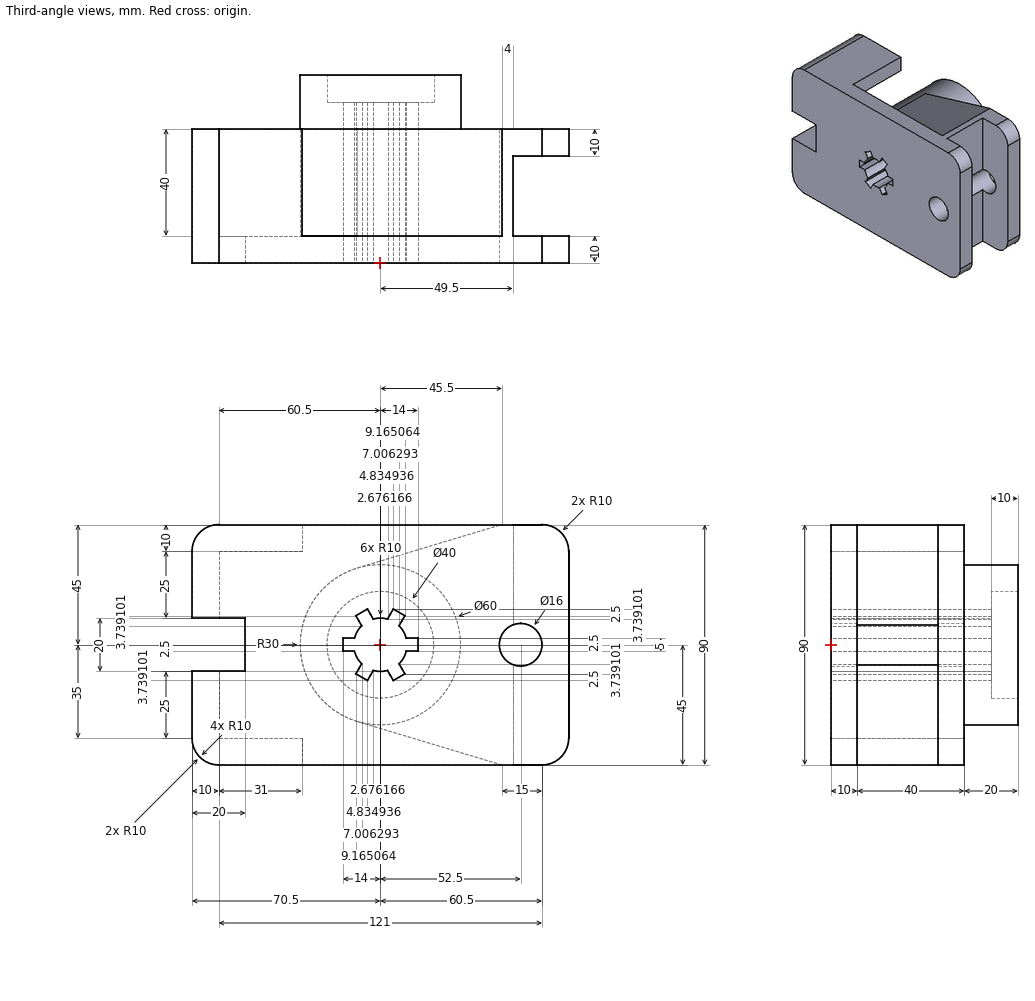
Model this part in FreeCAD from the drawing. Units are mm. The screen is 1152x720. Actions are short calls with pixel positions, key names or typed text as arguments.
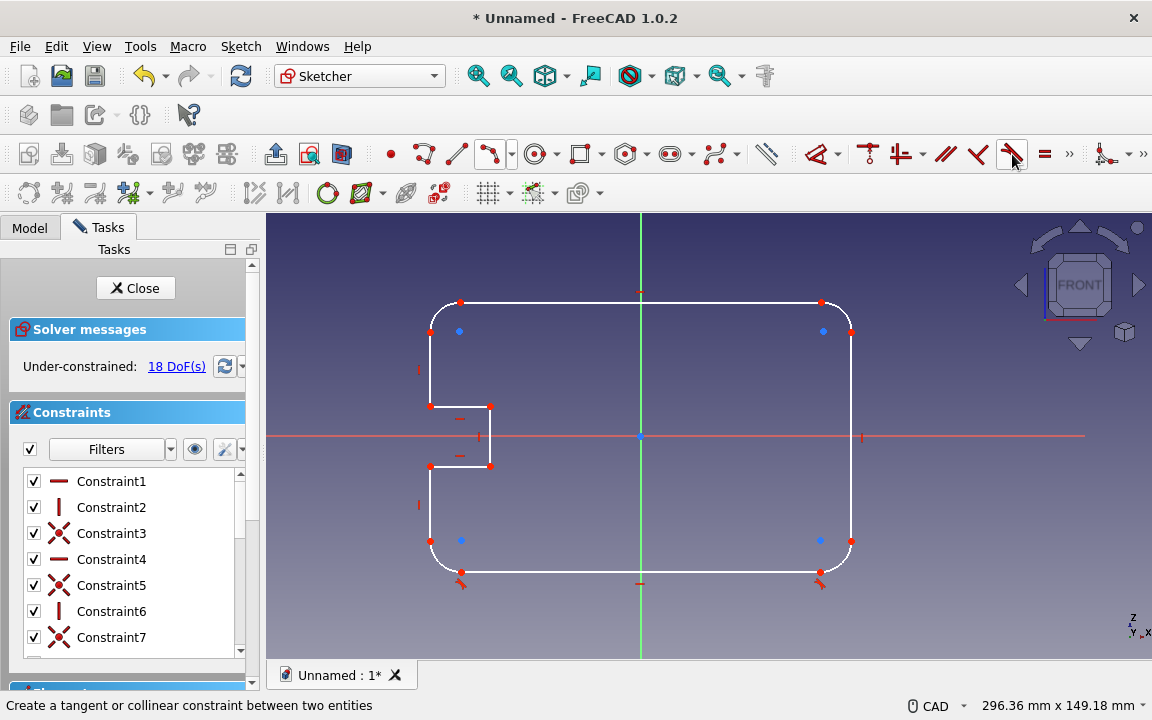
click(430, 519)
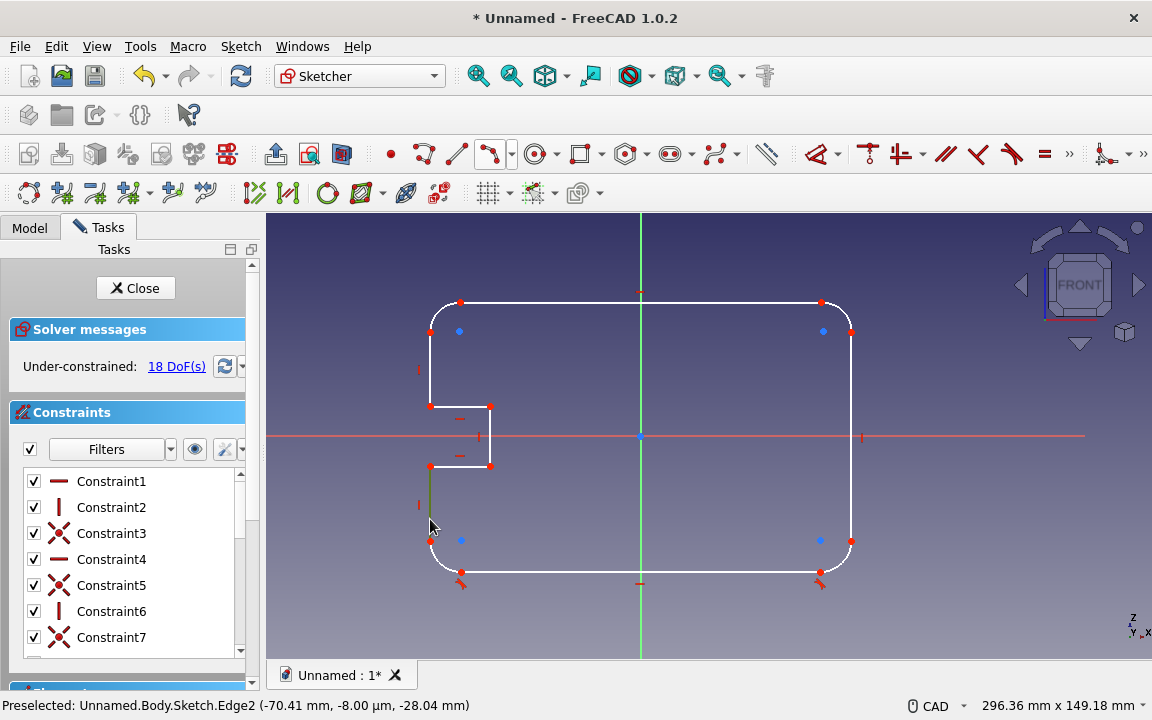
click(434, 556)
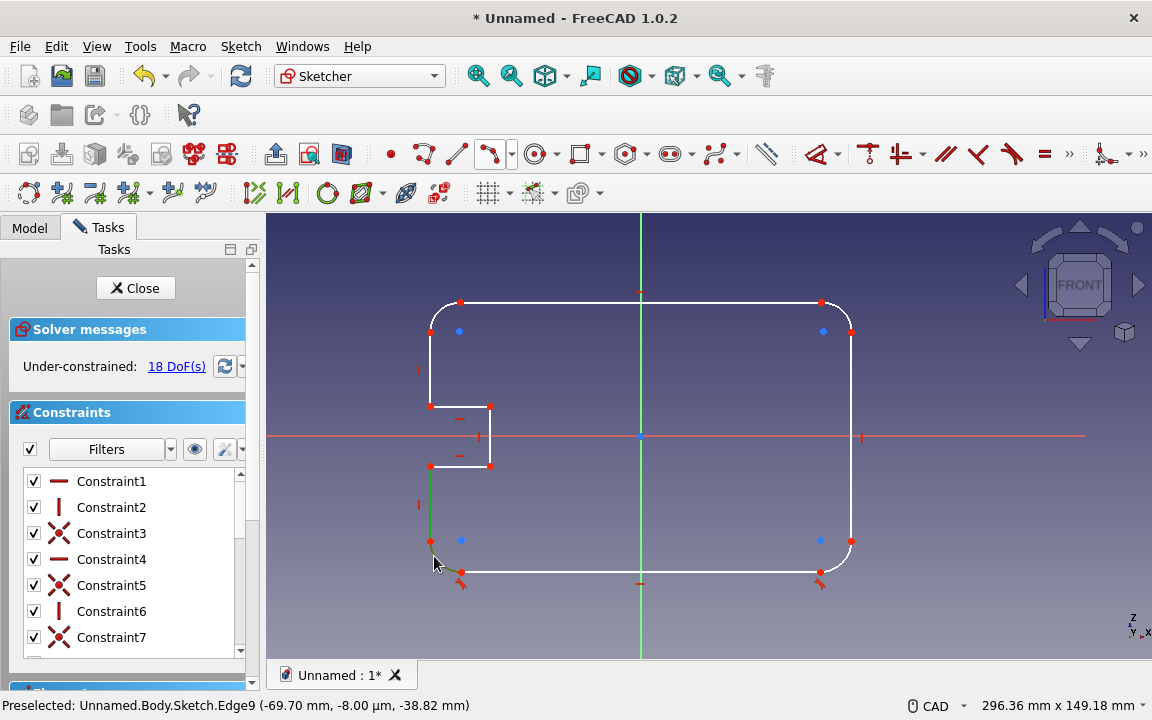
click(1012, 154)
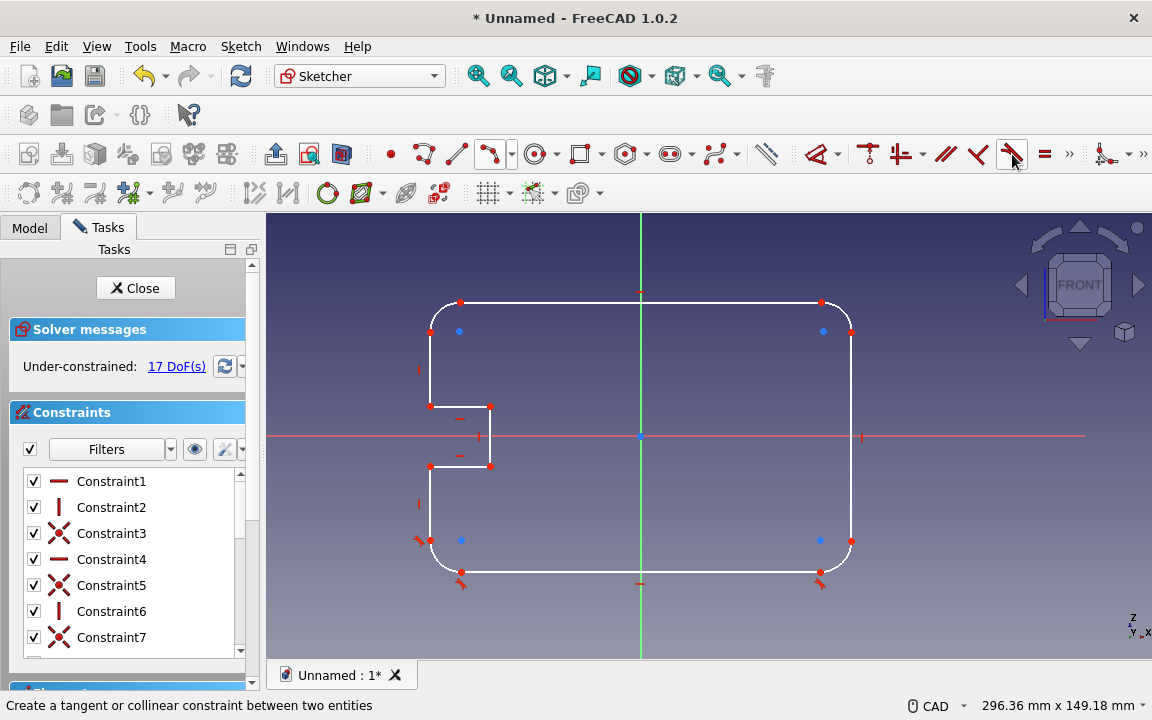
click(430, 385)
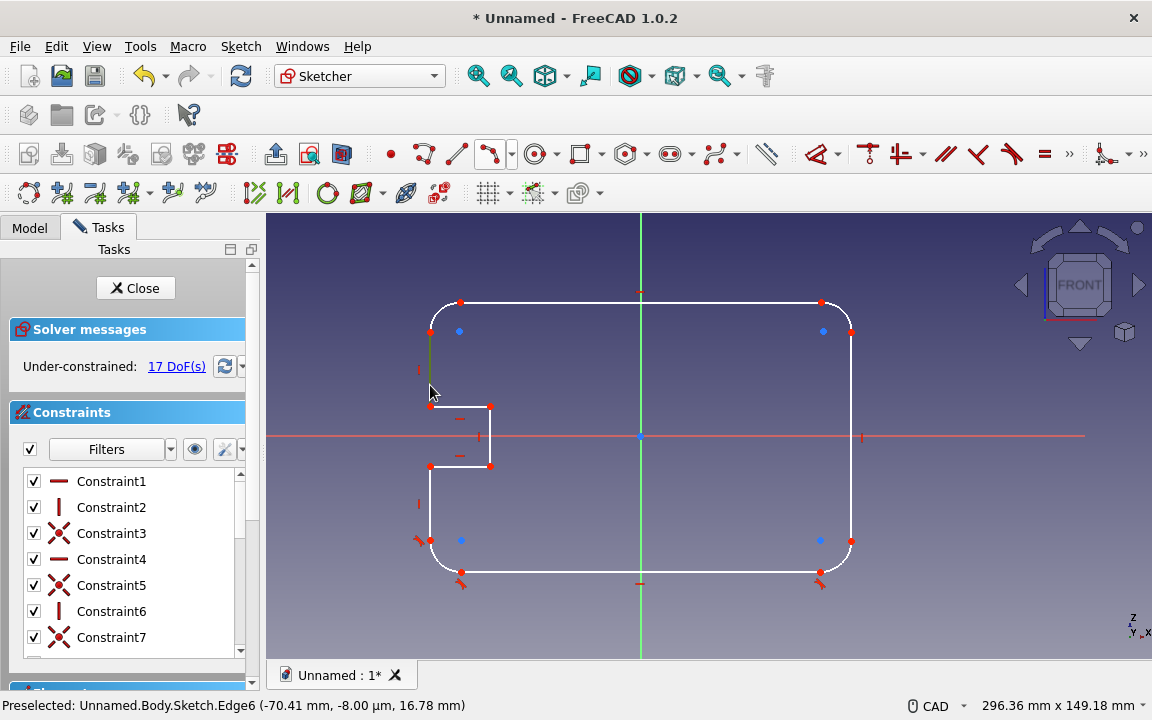
click(447, 306)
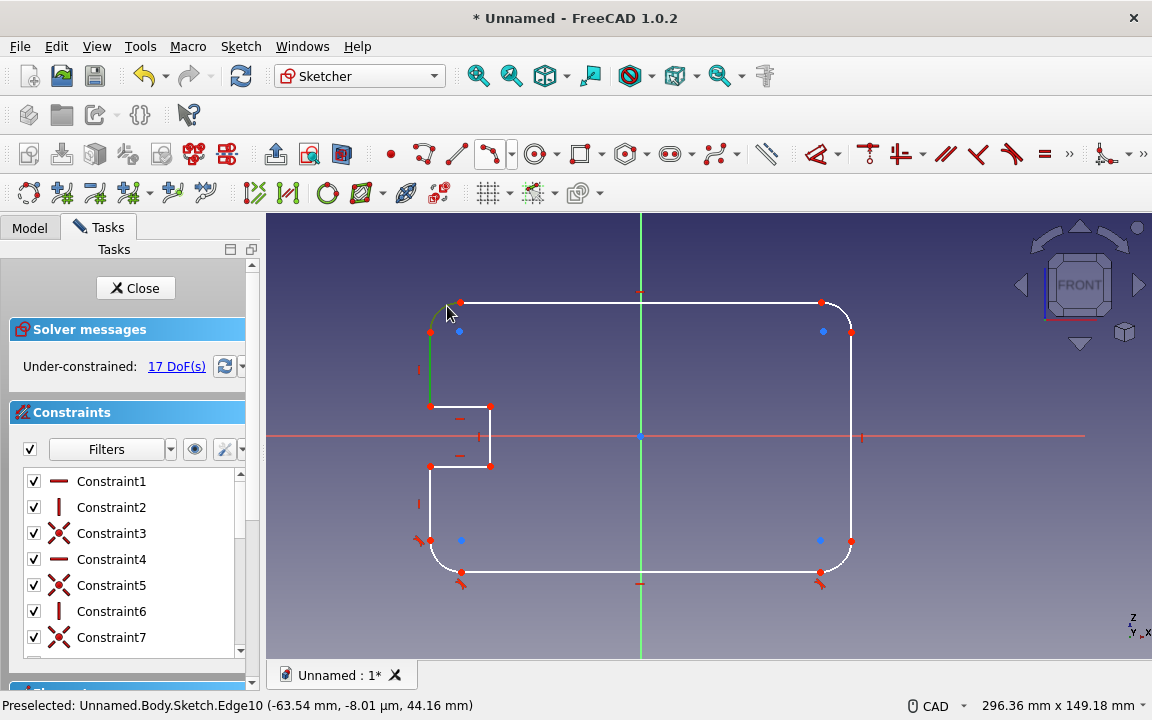
click(1012, 154)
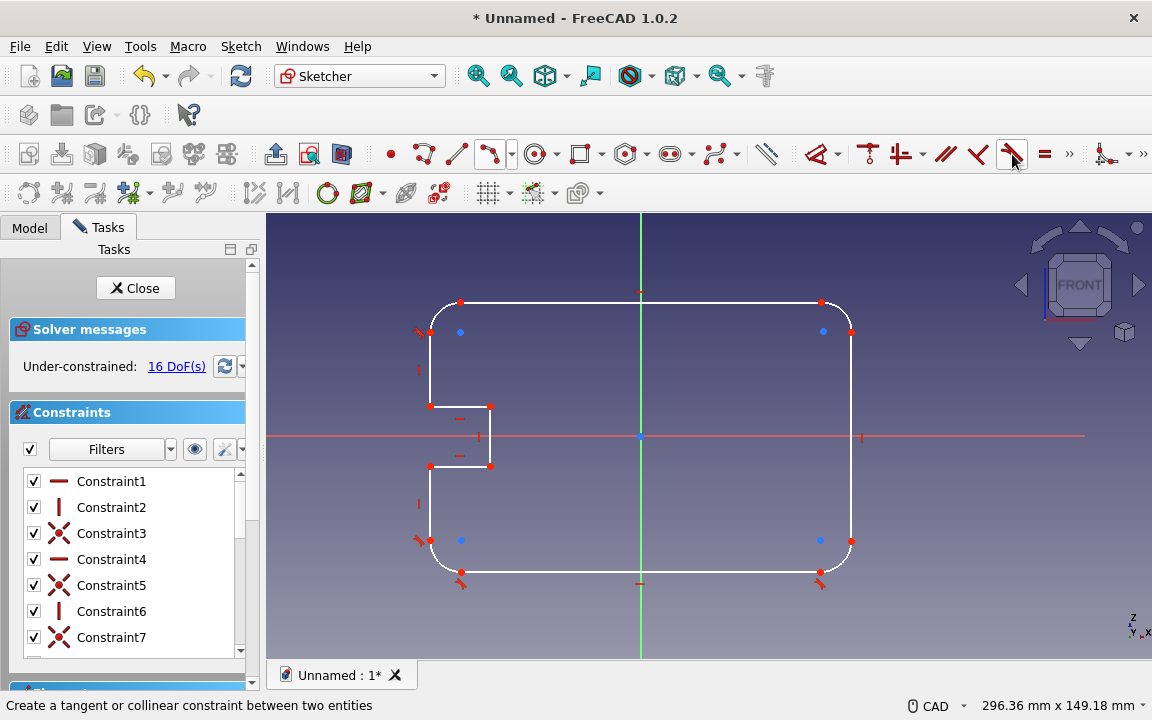
click(569, 303)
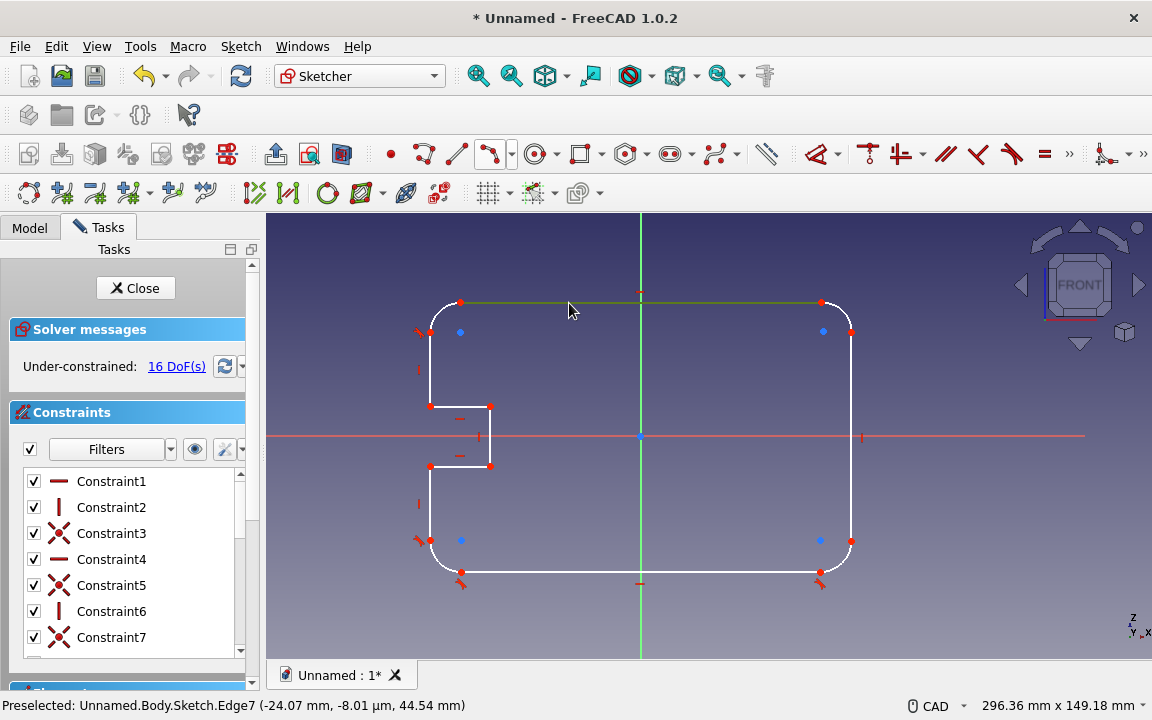
click(447, 306)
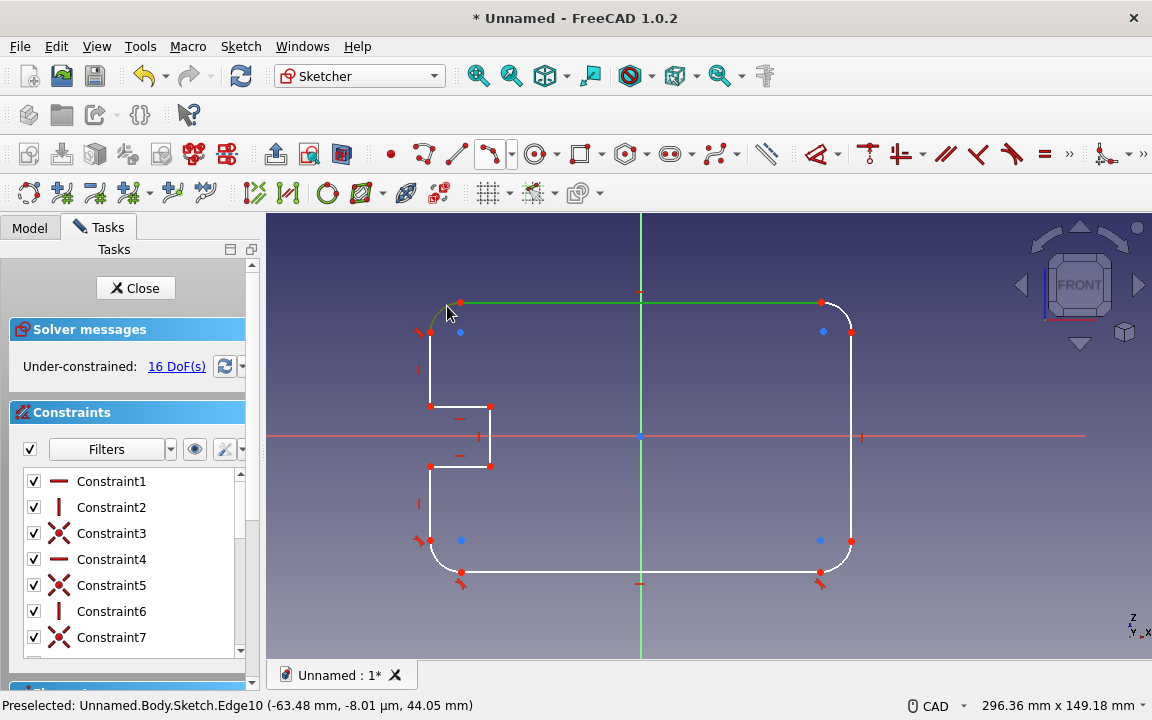
click(1012, 154)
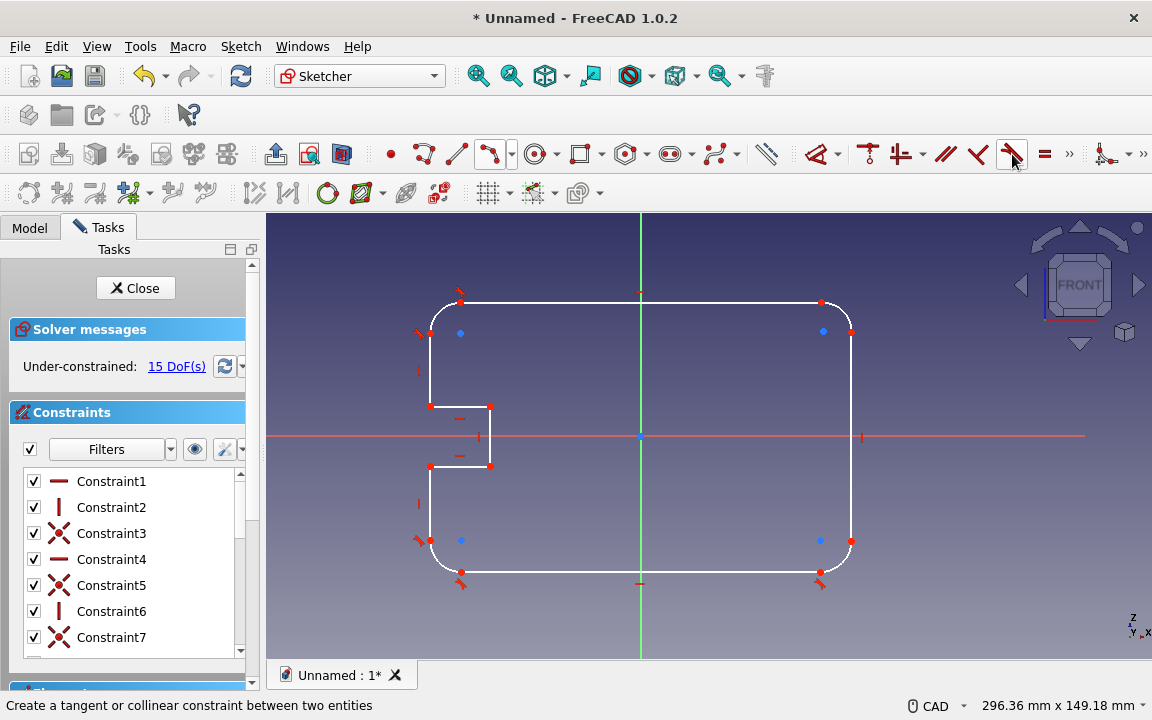
click(569, 303)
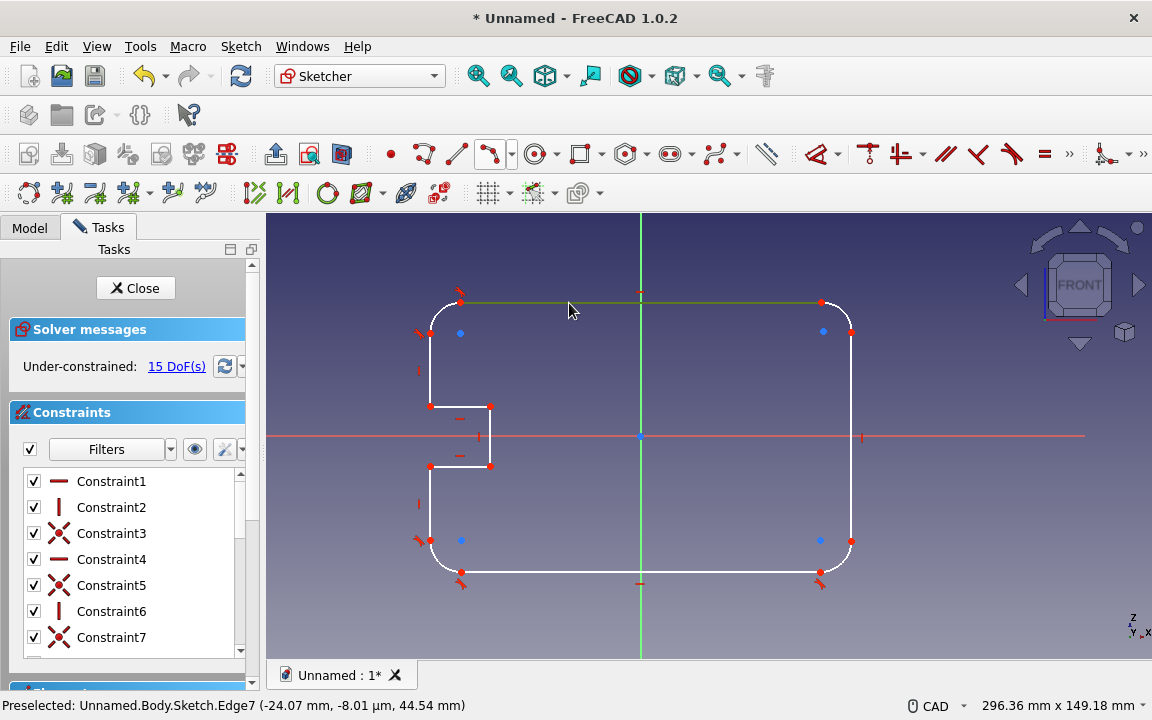
click(849, 319)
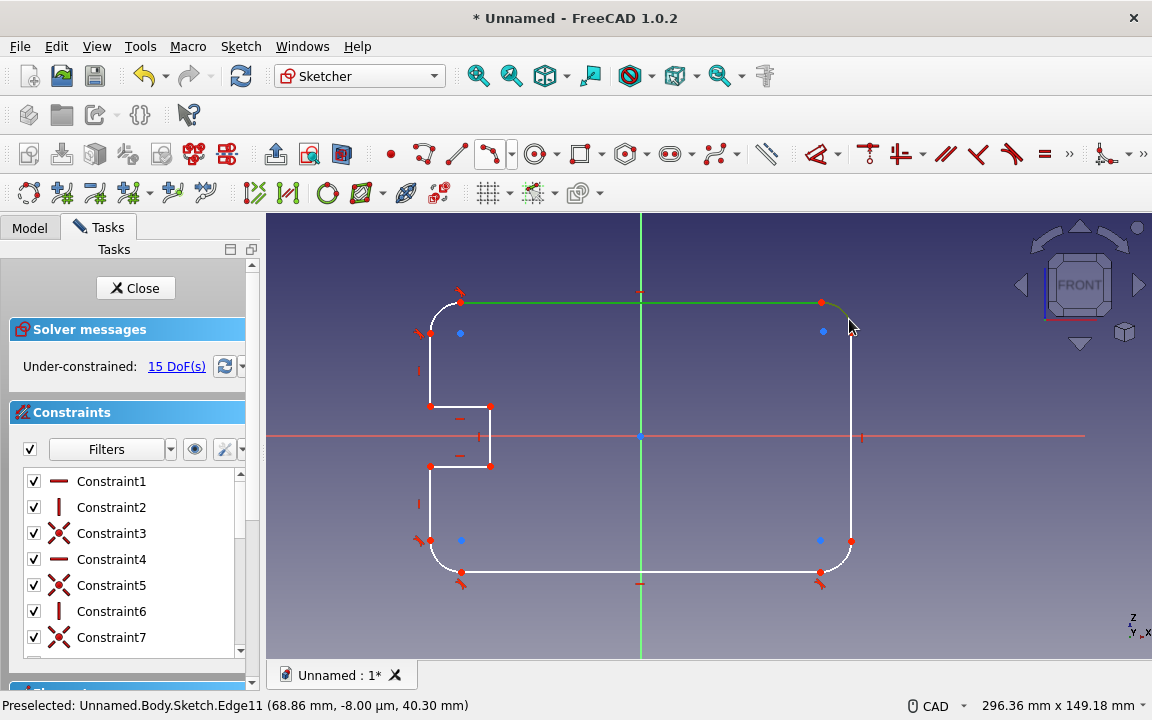
click(1012, 154)